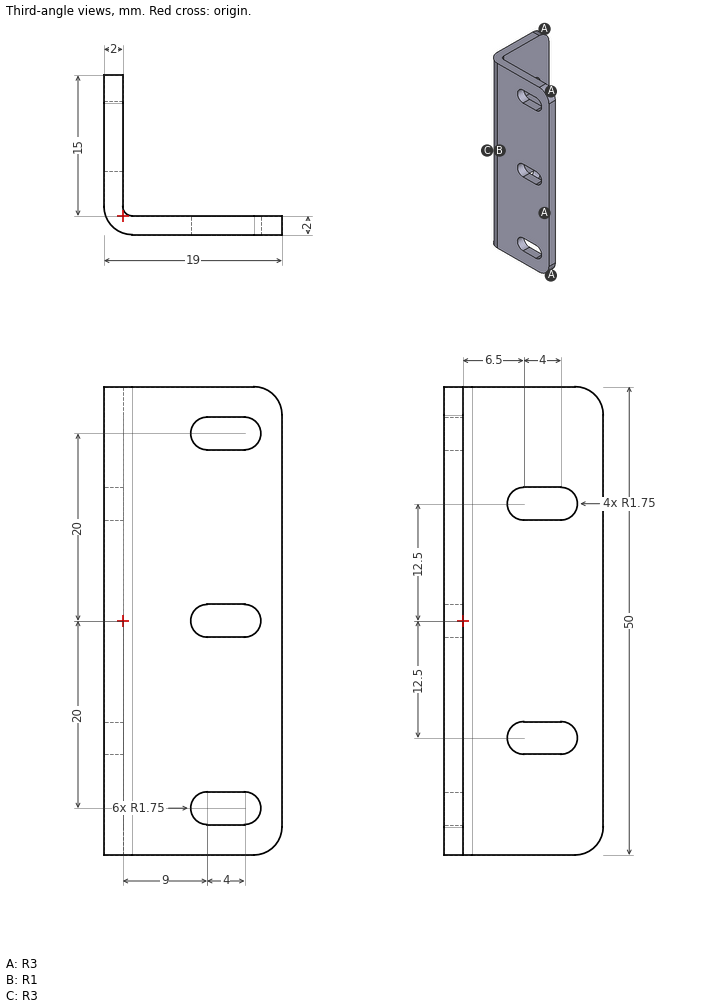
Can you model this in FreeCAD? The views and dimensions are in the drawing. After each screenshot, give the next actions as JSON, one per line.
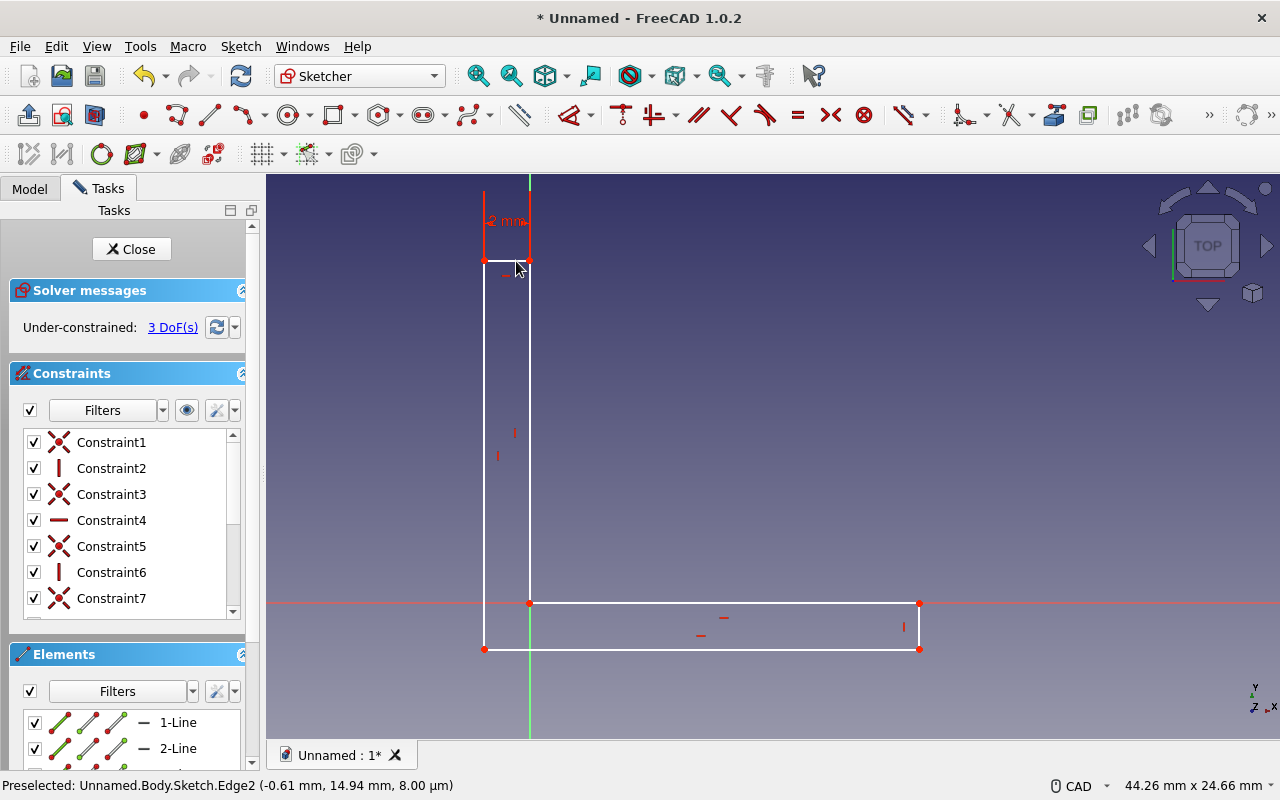
{"action": "left_click", "coordinate": [919, 636]}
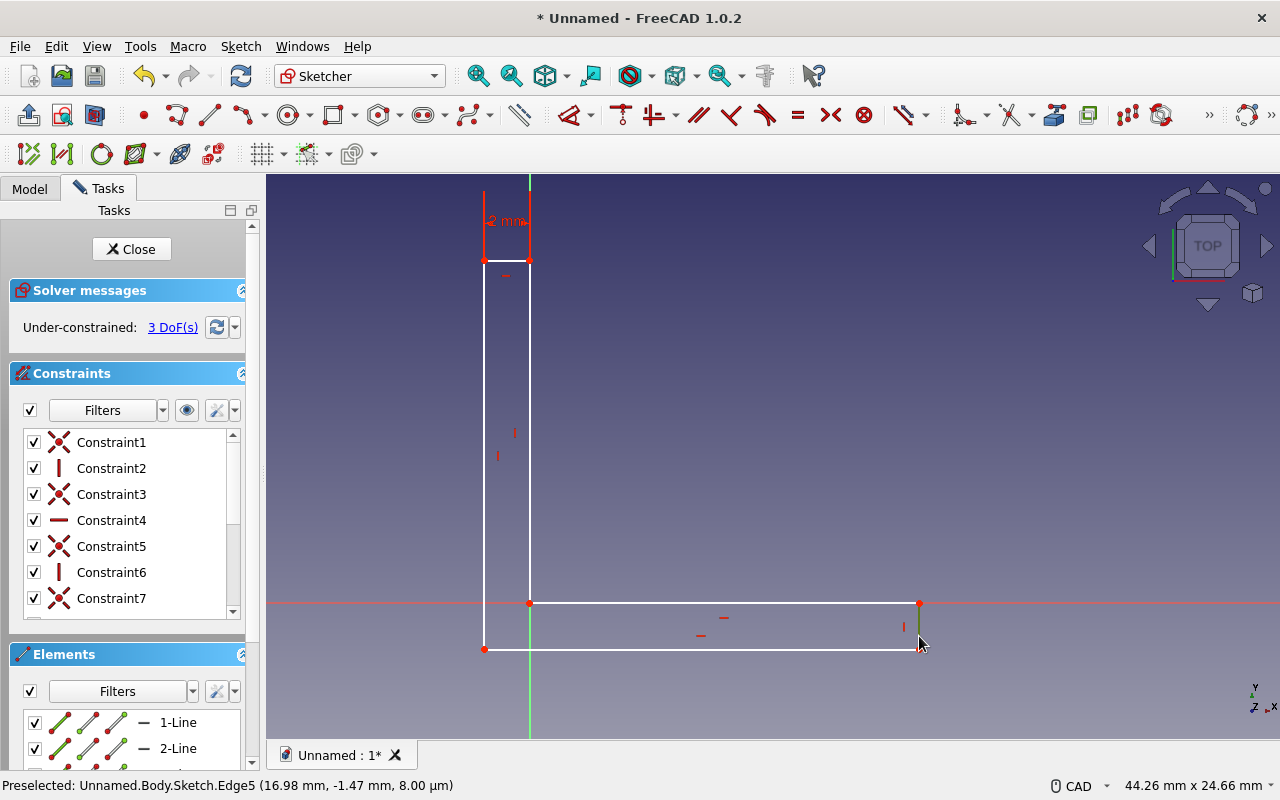
{"action": "left_click", "coordinate": [590, 116]}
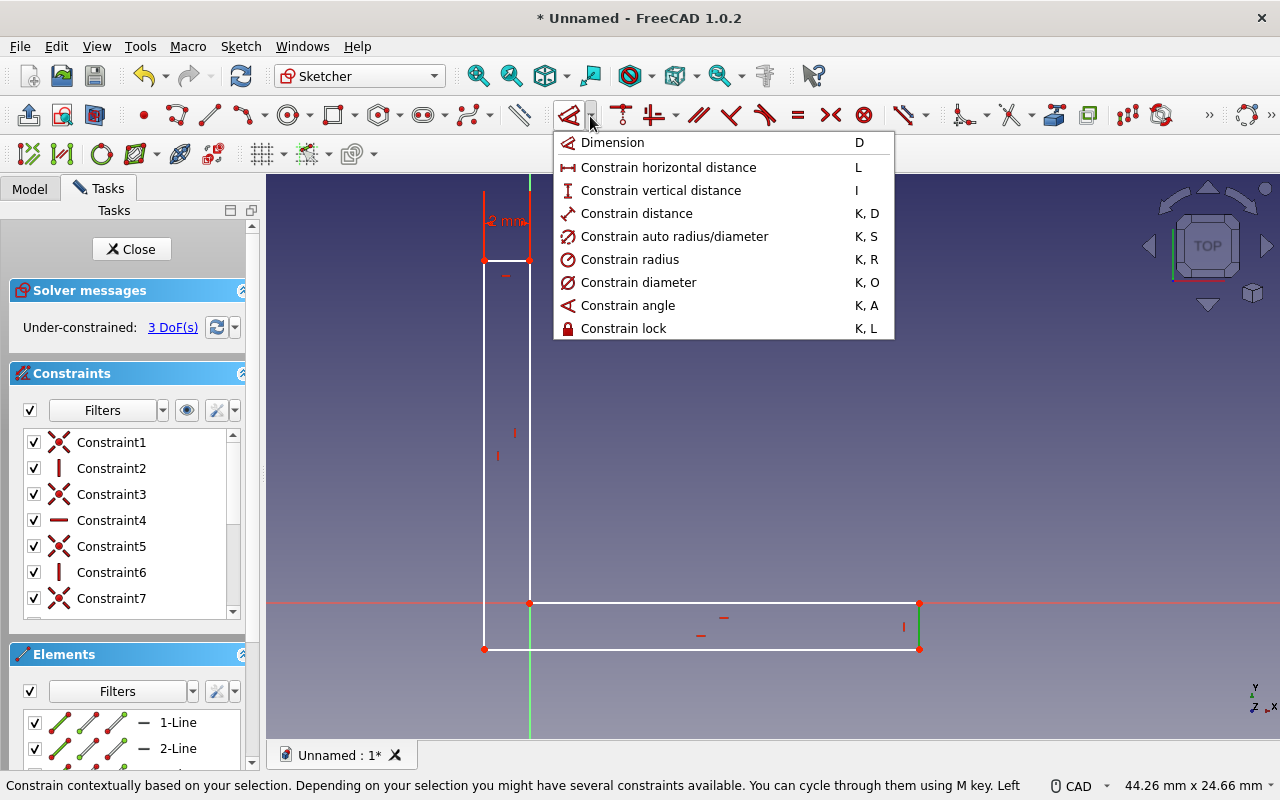
{"action": "left_click", "coordinate": [724, 190]}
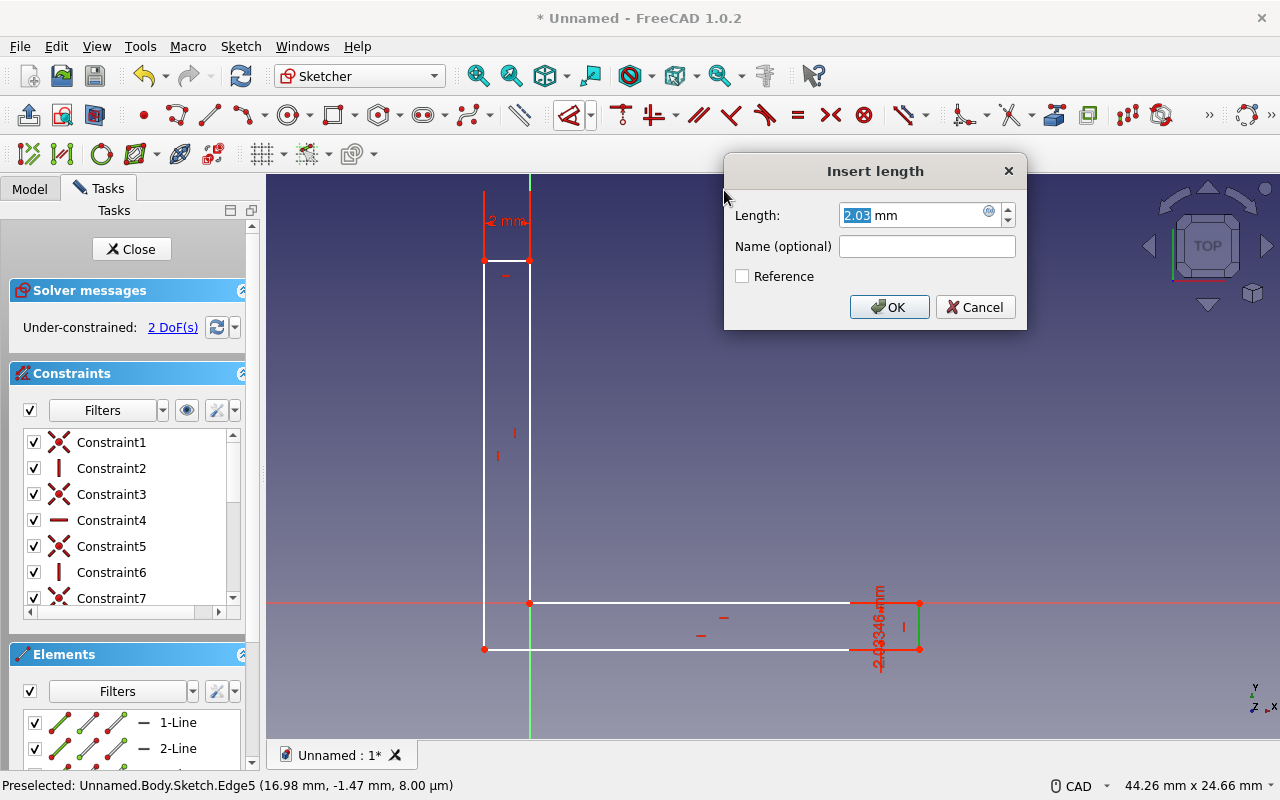
{"action": "type", "text": "2"}
{"action": "key", "text": "Return"}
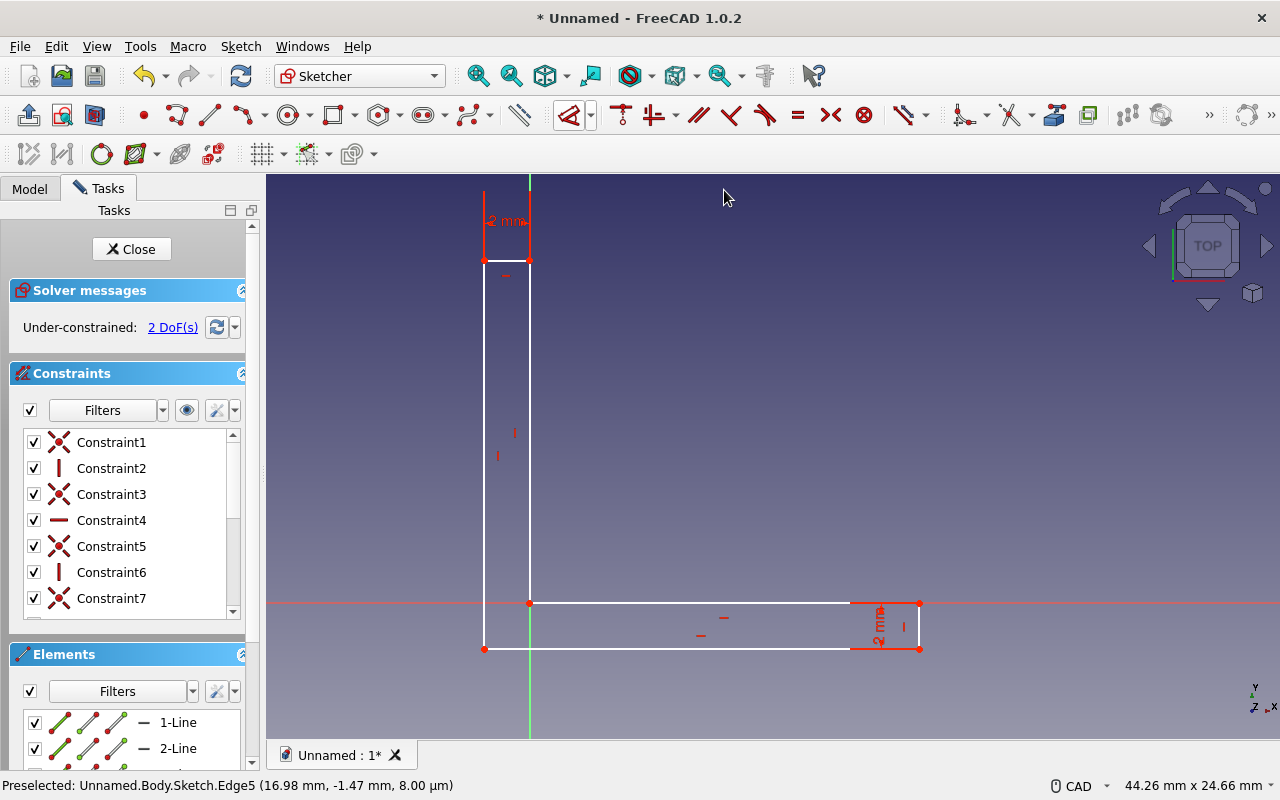
{"action": "left_click", "coordinate": [530, 501]}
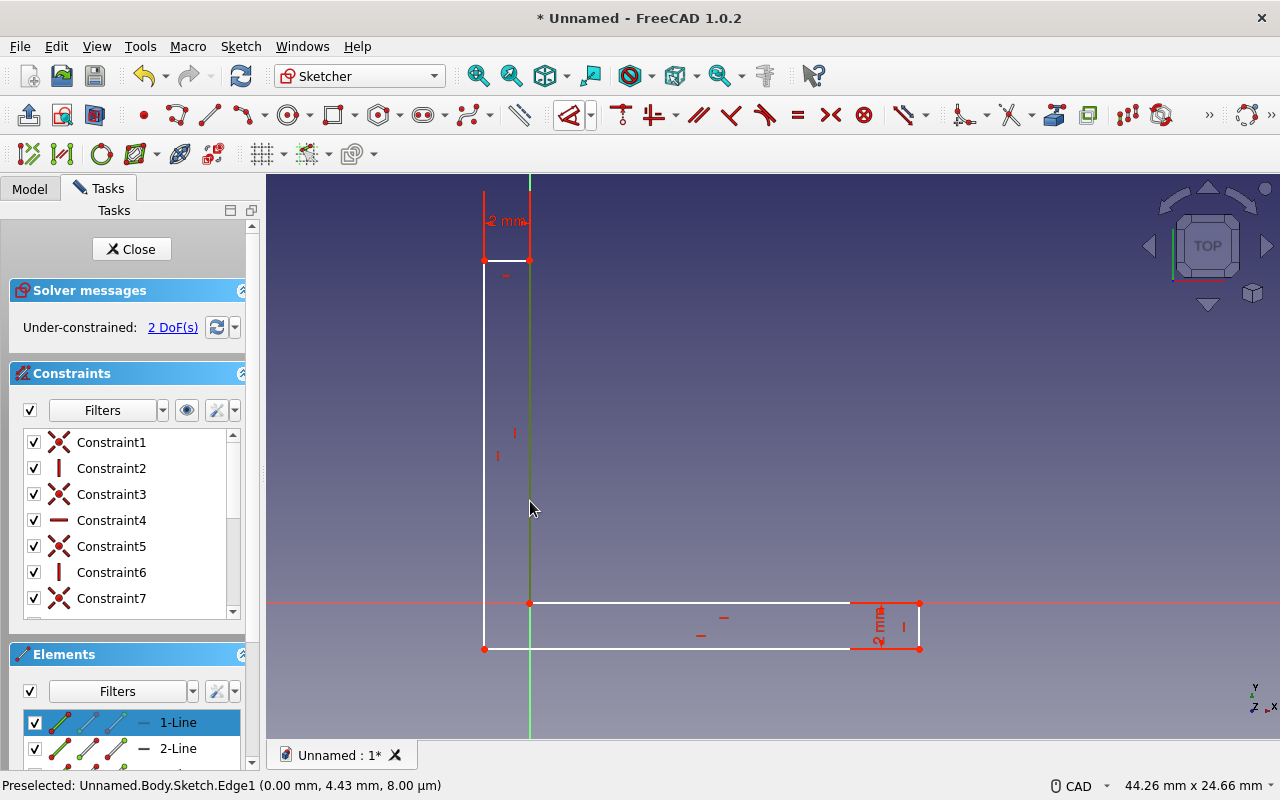
{"action": "key", "text": "i"}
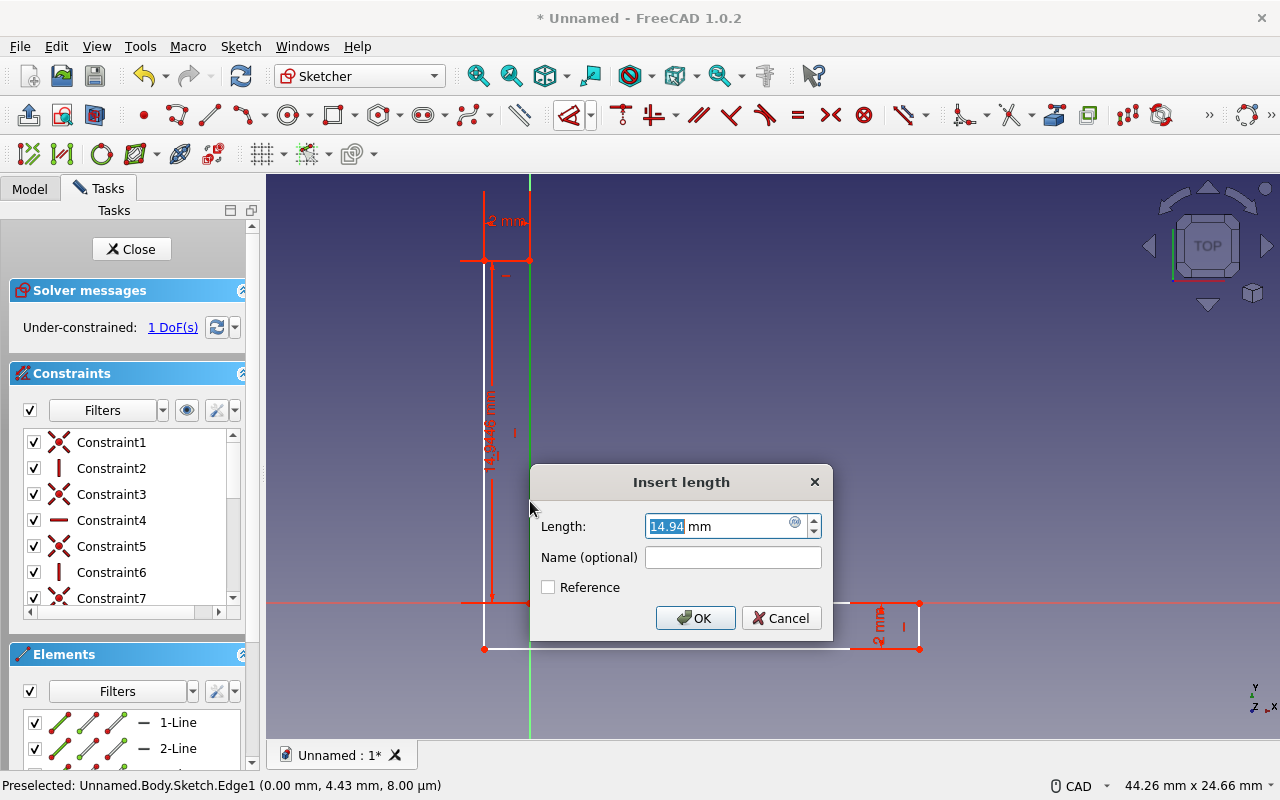
{"action": "type", "text": "15"}
{"action": "key", "text": "Return"}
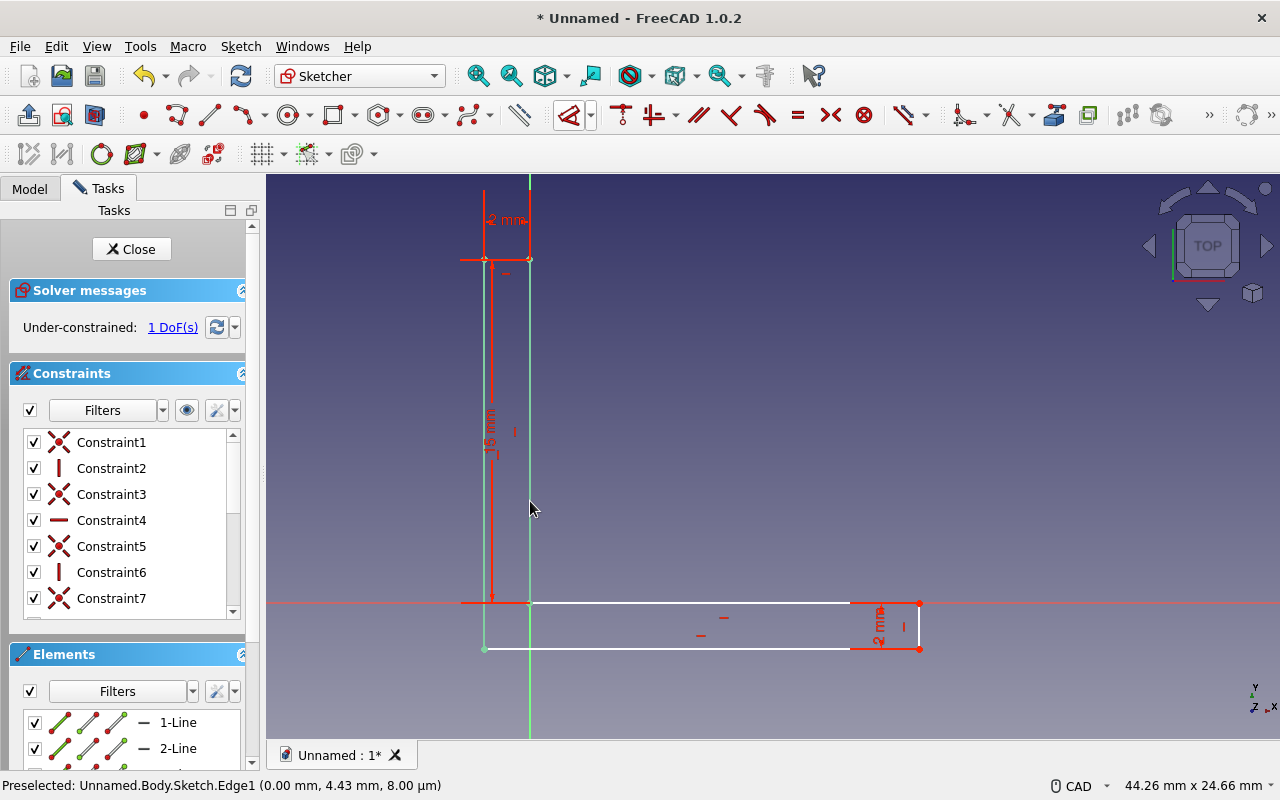
{"action": "left_click", "coordinate": [615, 649]}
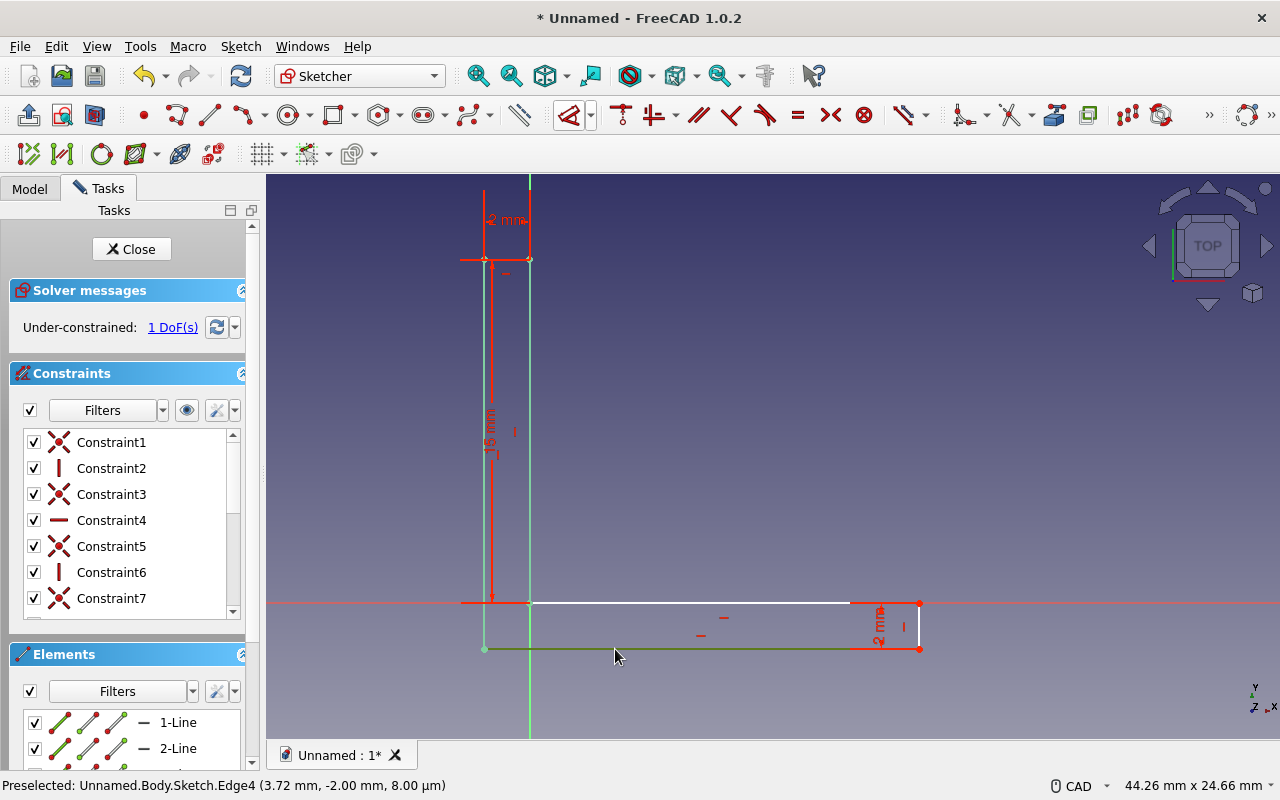
{"action": "left_click", "coordinate": [590, 116]}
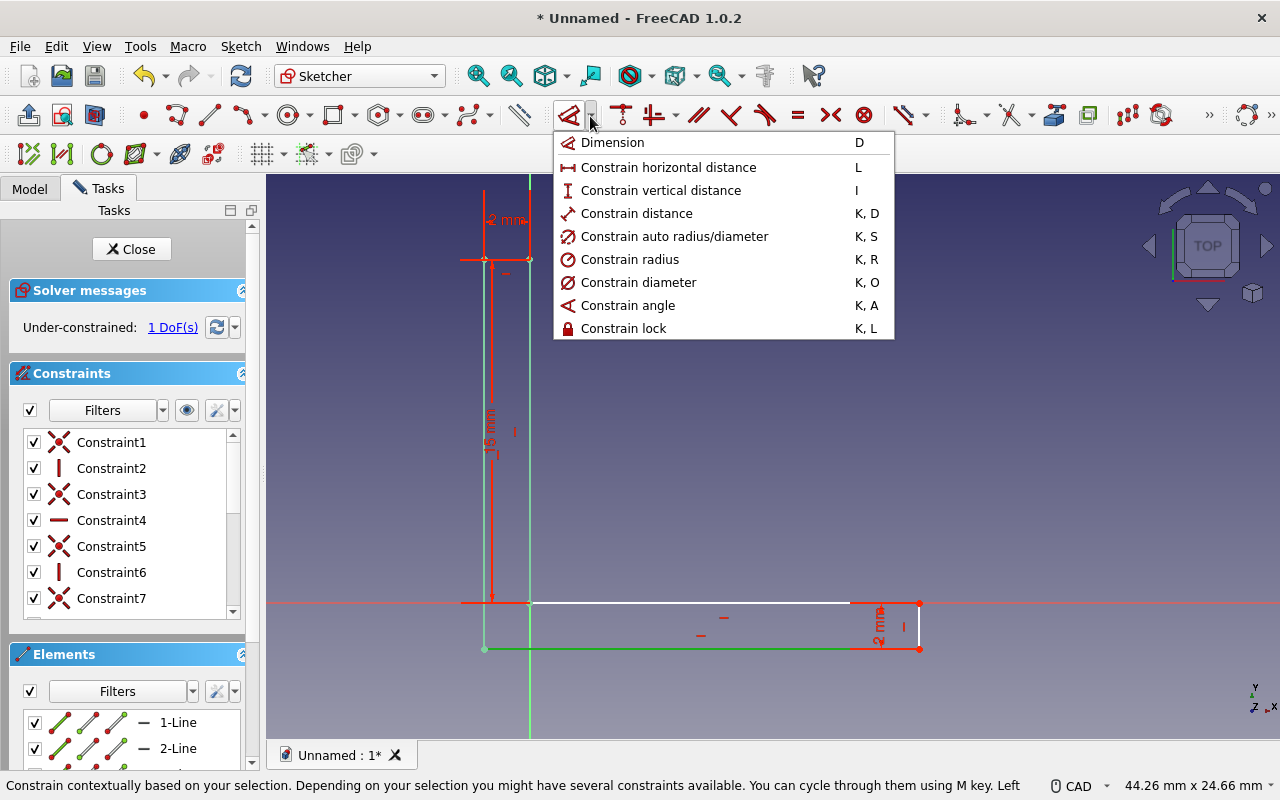
{"action": "left_click", "coordinate": [724, 168]}